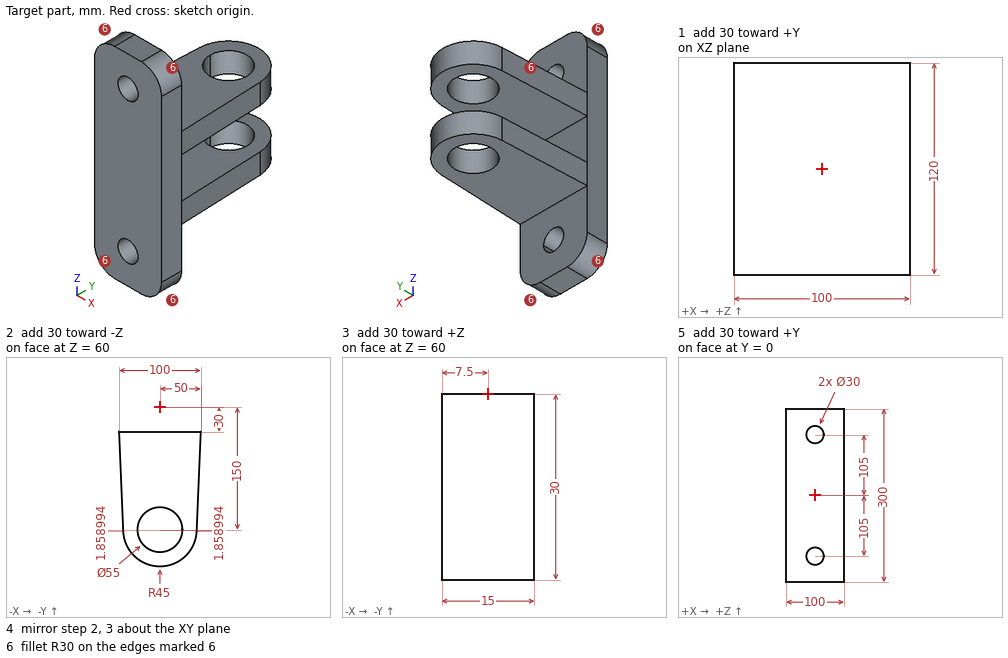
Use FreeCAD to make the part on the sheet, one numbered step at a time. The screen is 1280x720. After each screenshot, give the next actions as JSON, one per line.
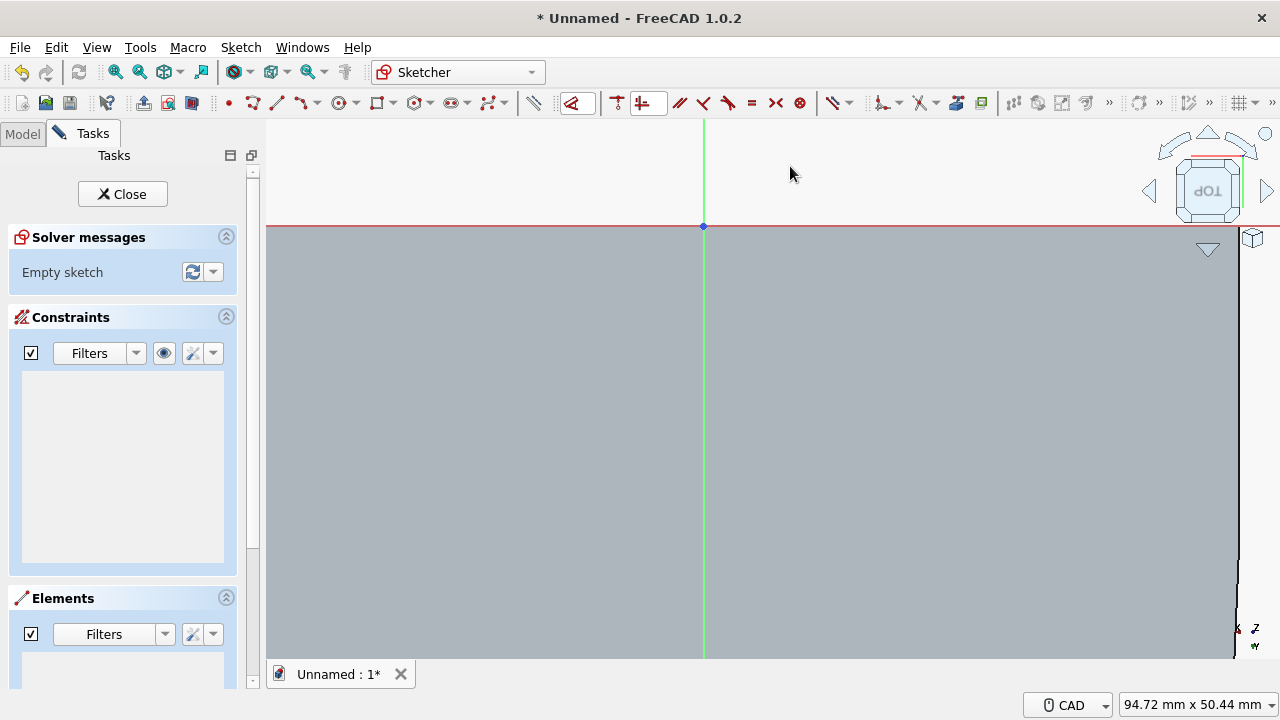
{"action": "left_click", "coordinate": [378, 104]}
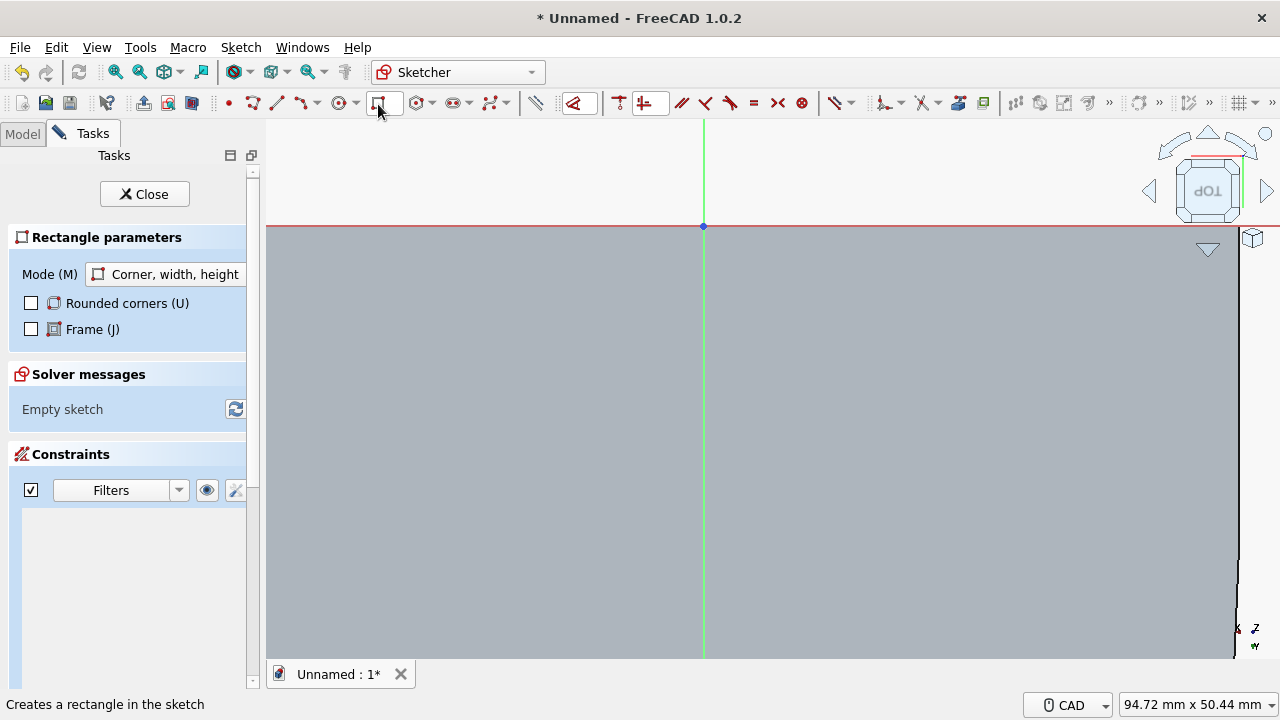
{"action": "left_click", "coordinate": [623, 226]}
{"action": "mouse_move", "coordinate": [784, 548]}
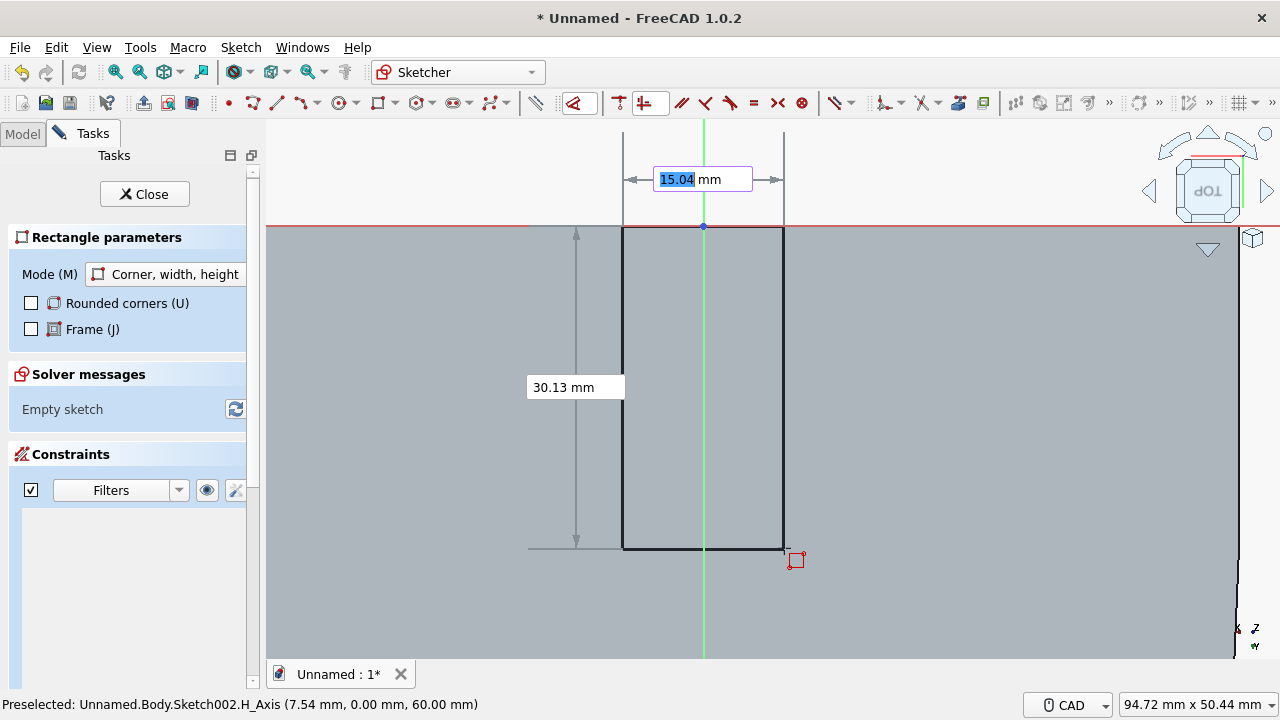
{"action": "type", "text": "15"}
{"action": "key", "text": "Tab"}
{"action": "type", "text": "30"}
{"action": "key", "text": "Return"}
{"action": "key", "text": "Escape"}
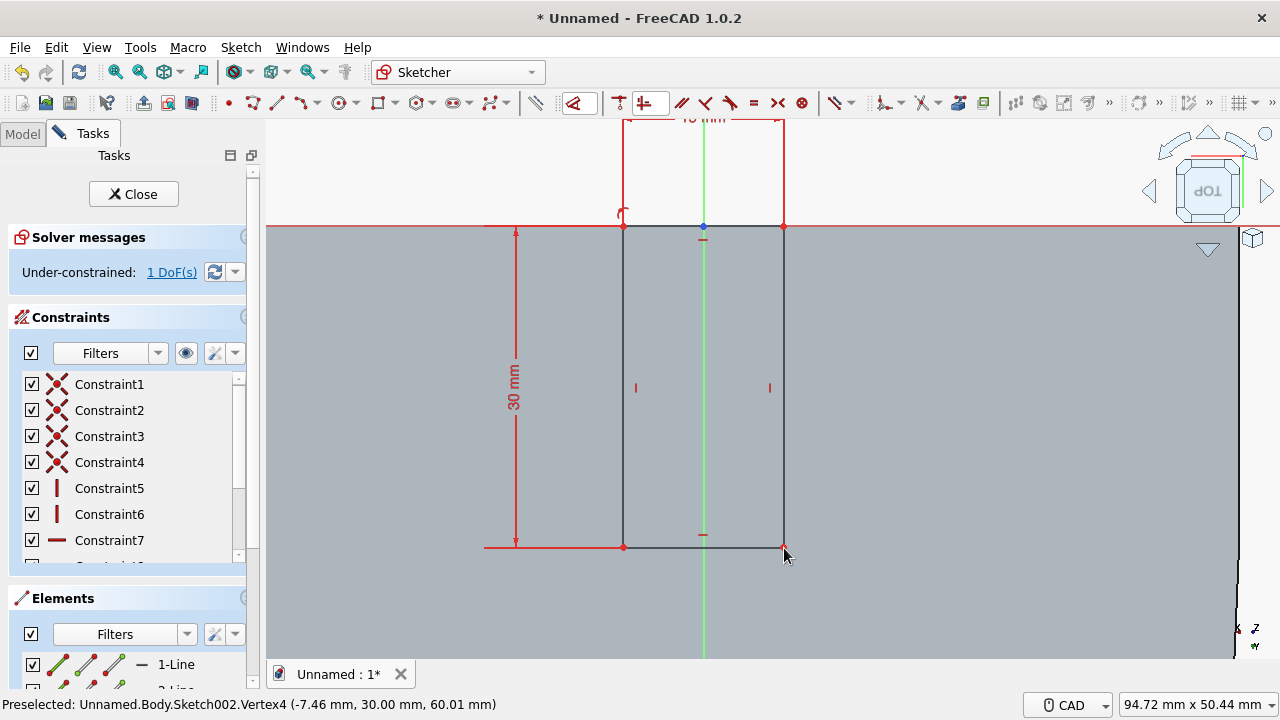
{"action": "left_click", "coordinate": [623, 226]}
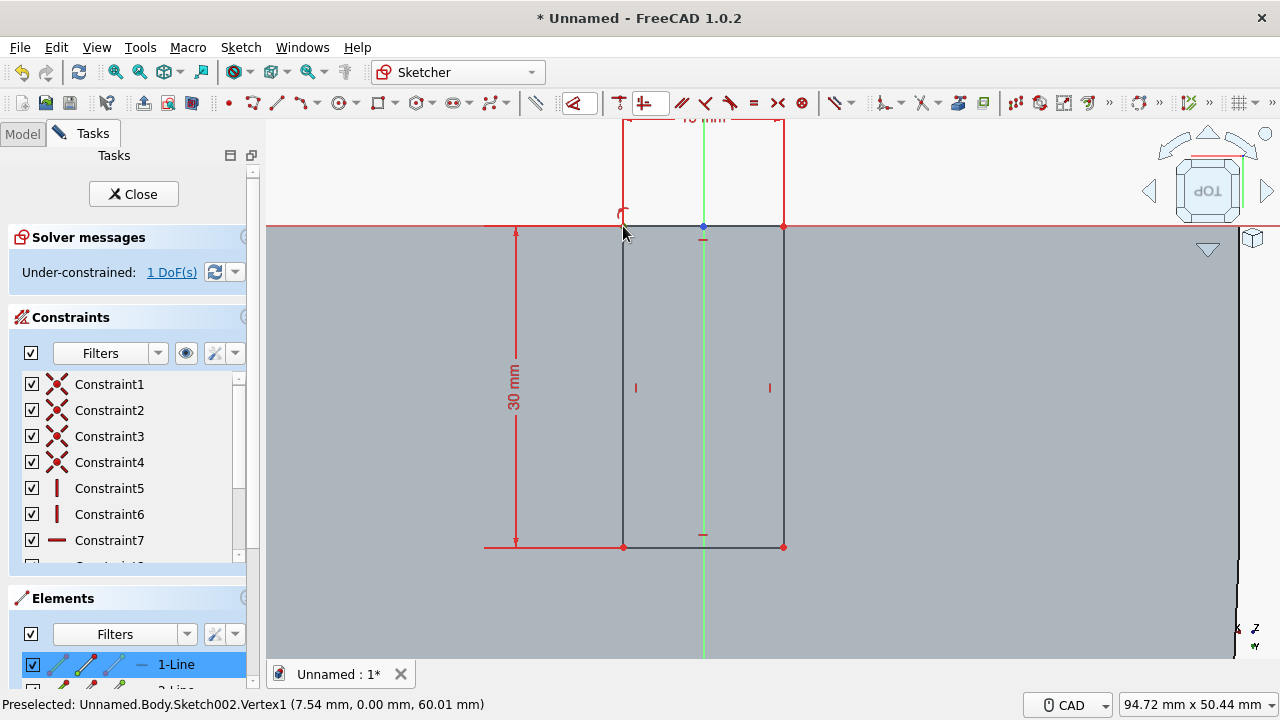
{"action": "left_click", "coordinate": [592, 104]}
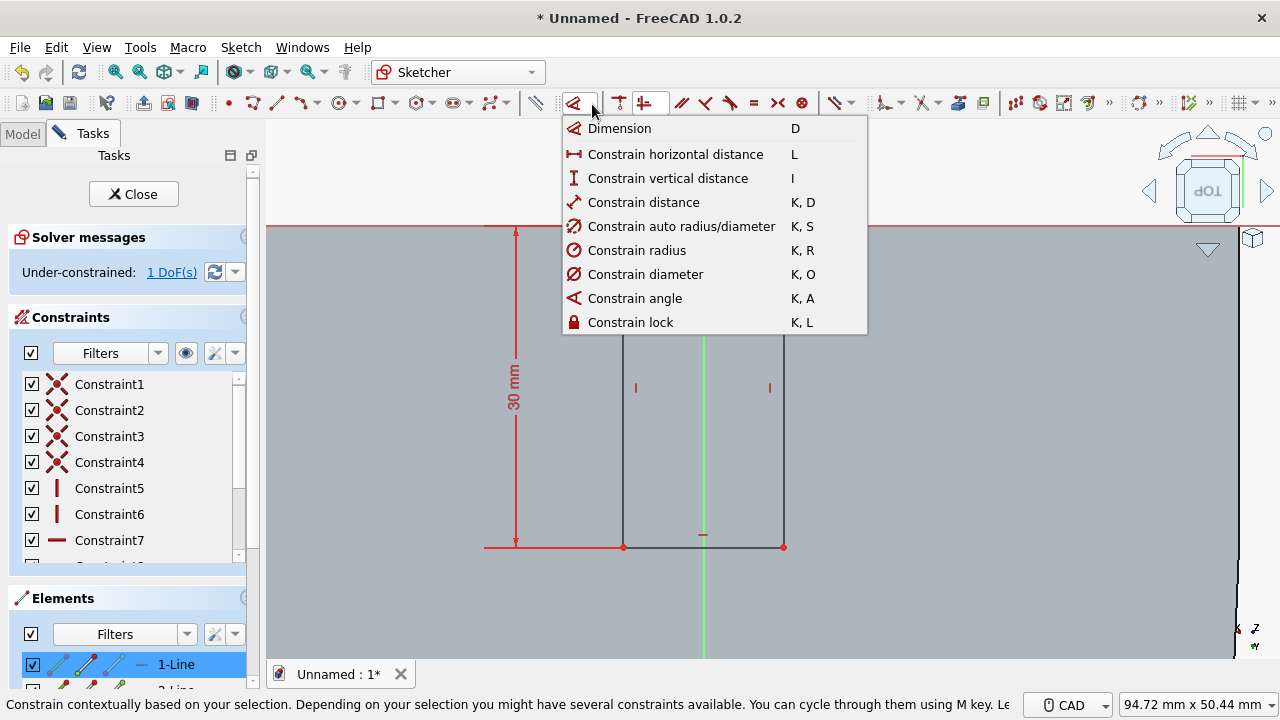
{"action": "left_click", "coordinate": [715, 154]}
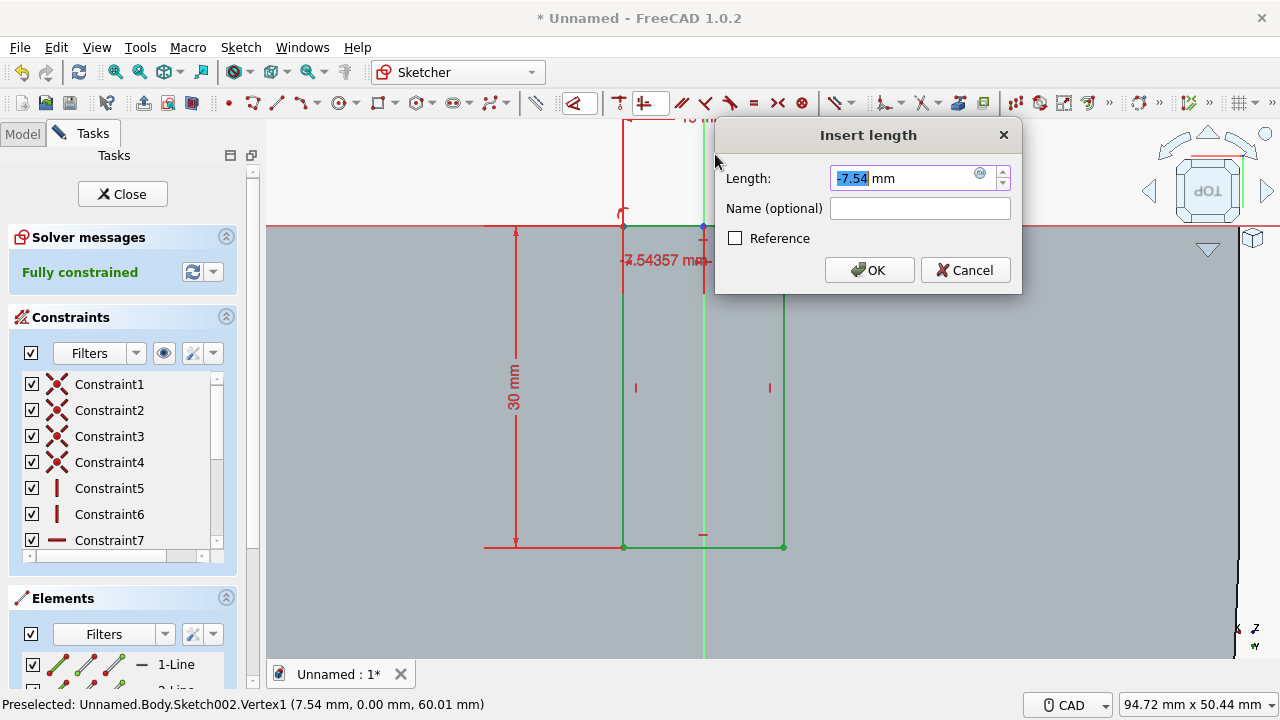
{"action": "type", "text": "-7.5"}
{"action": "key", "text": "Return"}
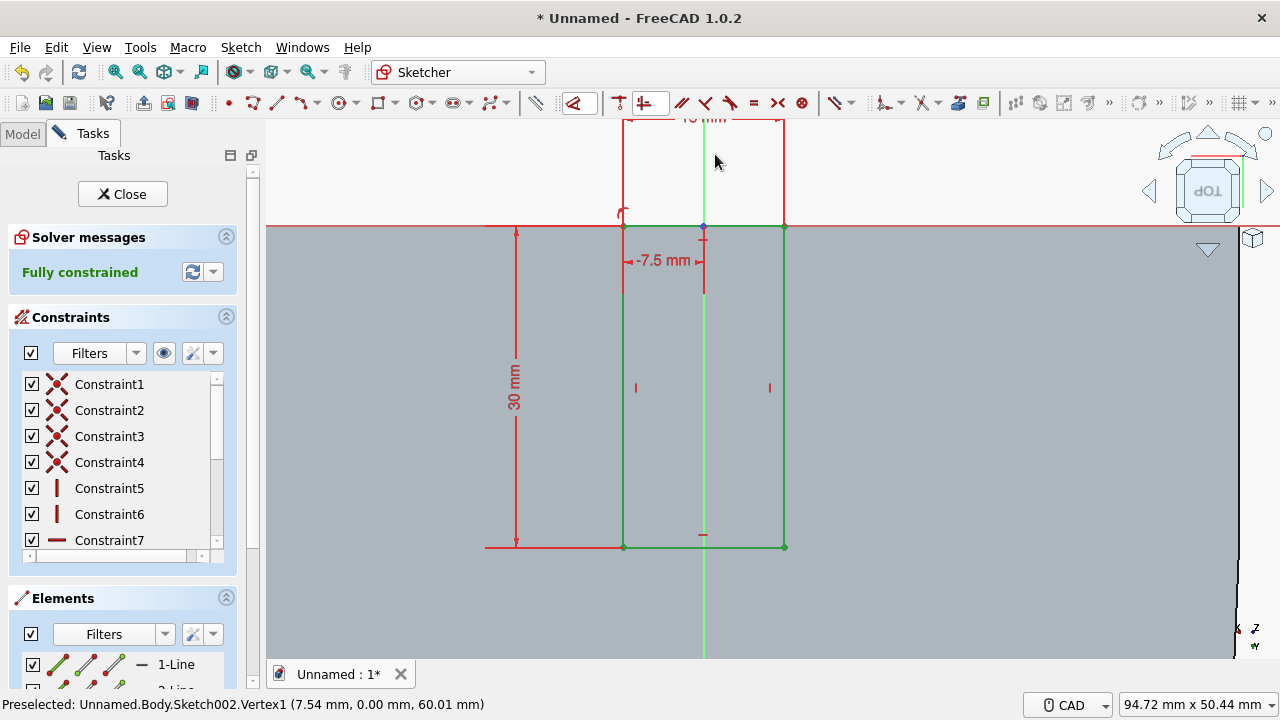
{"action": "left_click", "coordinate": [123, 194]}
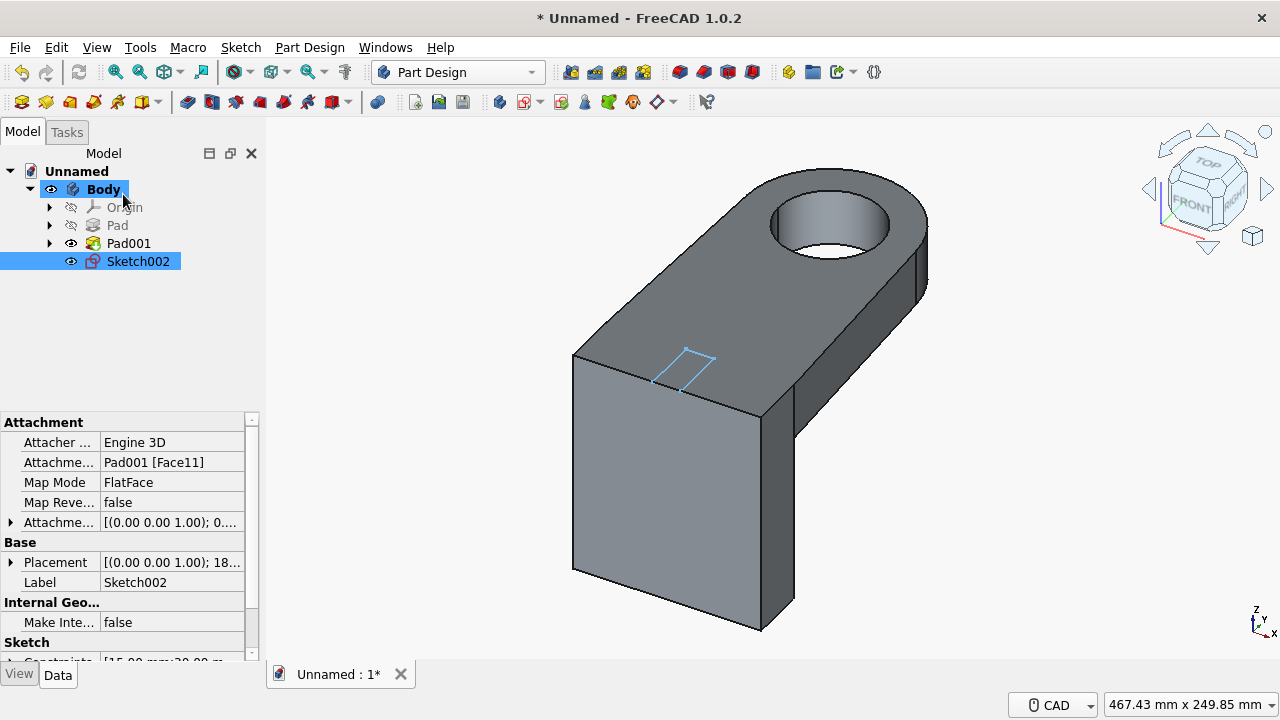
{"action": "left_click", "coordinate": [22, 102]}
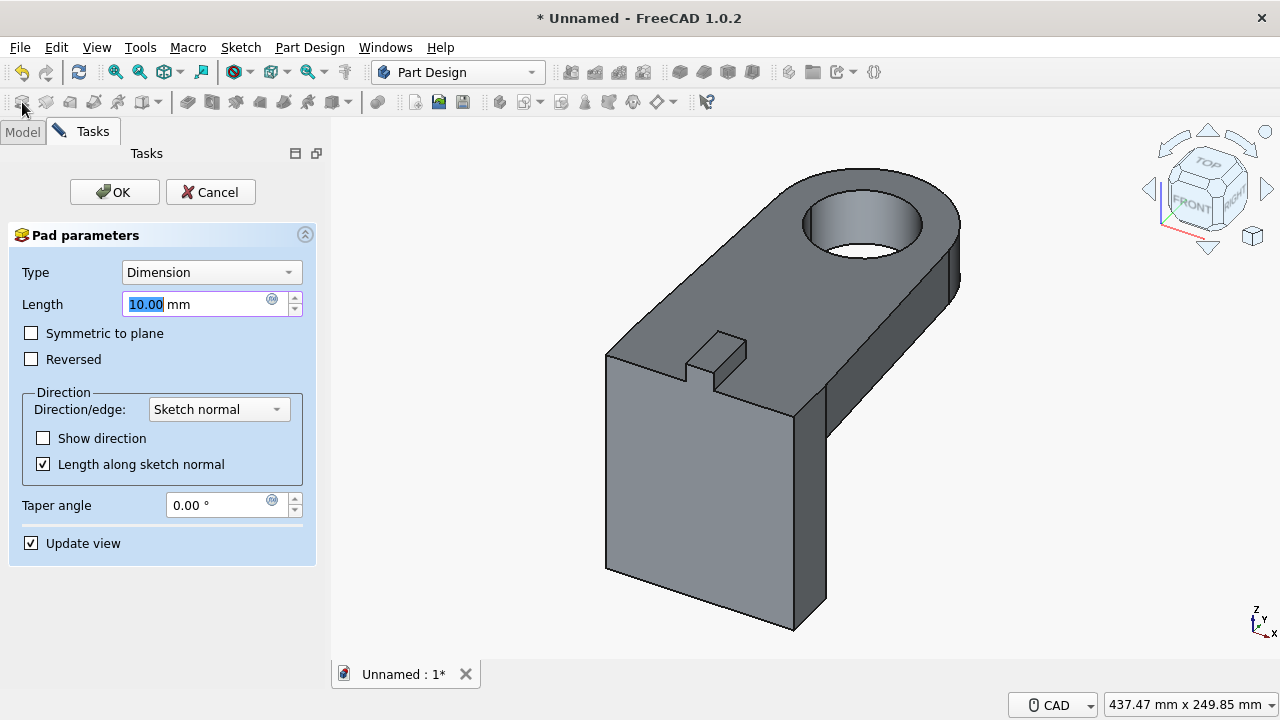
{"action": "type", "text": "30"}
{"action": "key", "text": "Tab"}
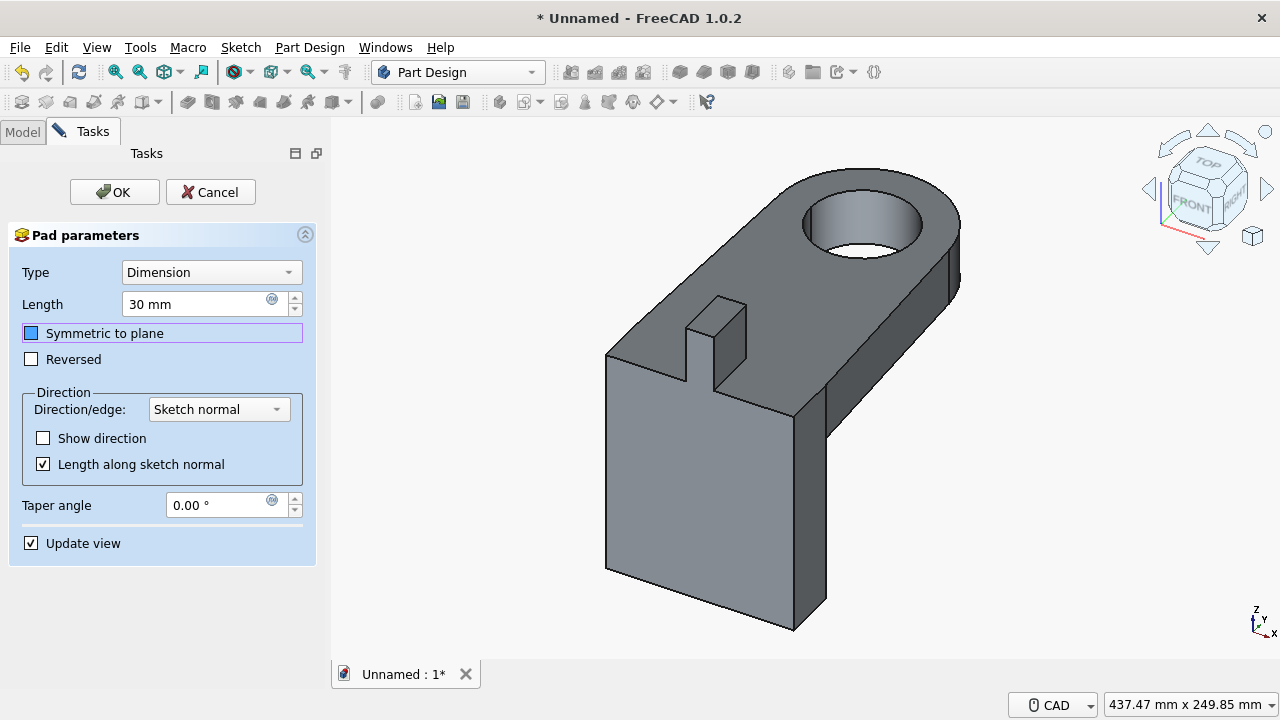
{"action": "left_click", "coordinate": [115, 192]}